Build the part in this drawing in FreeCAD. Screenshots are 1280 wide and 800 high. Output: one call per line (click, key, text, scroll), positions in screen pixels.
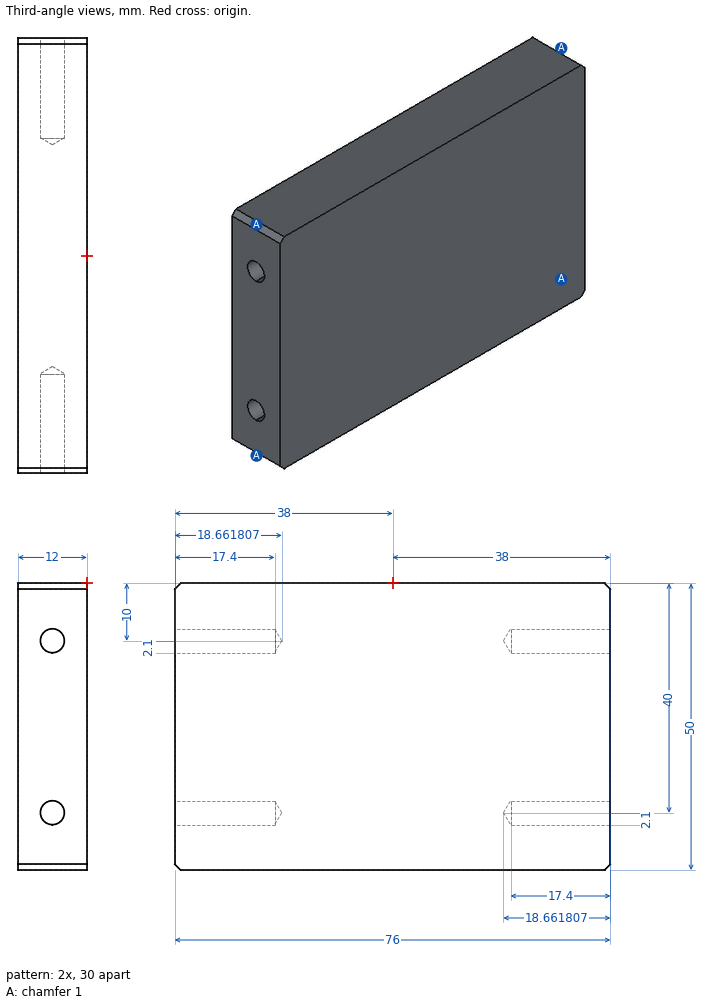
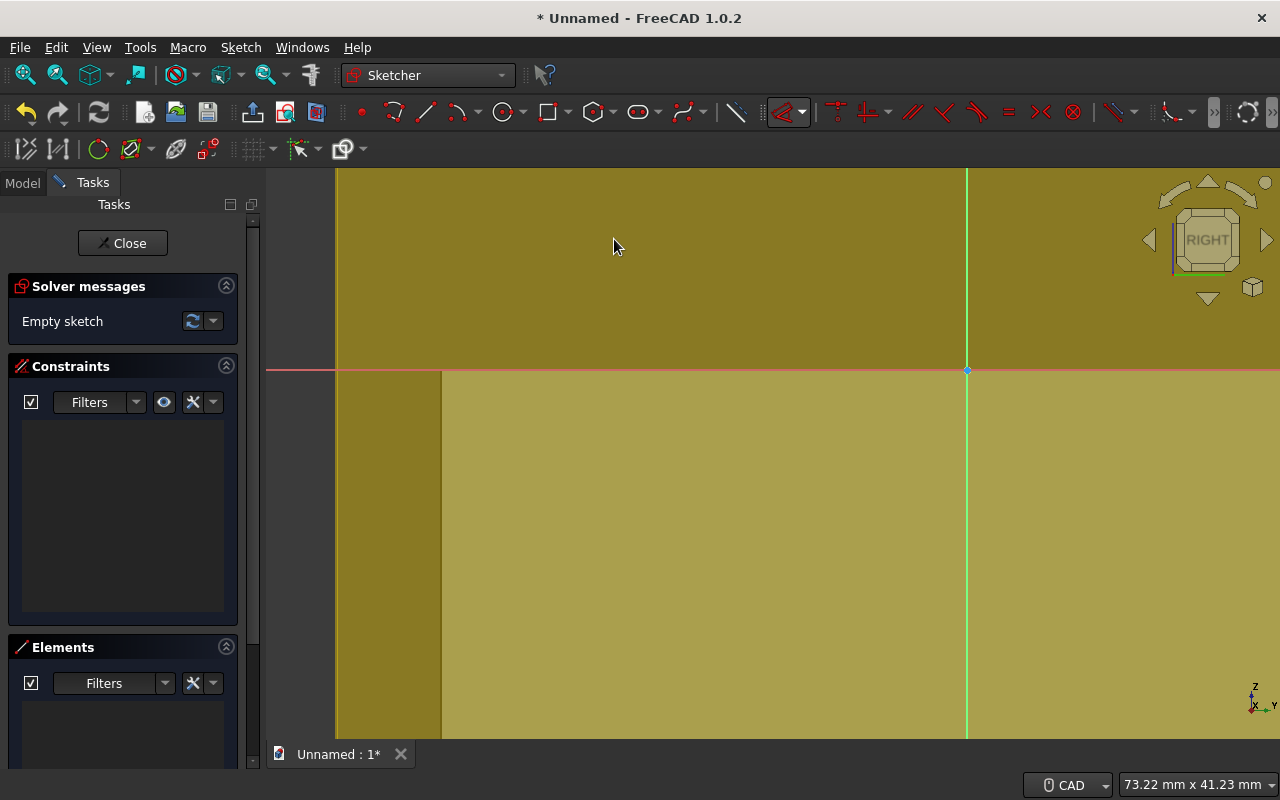
click(394, 112)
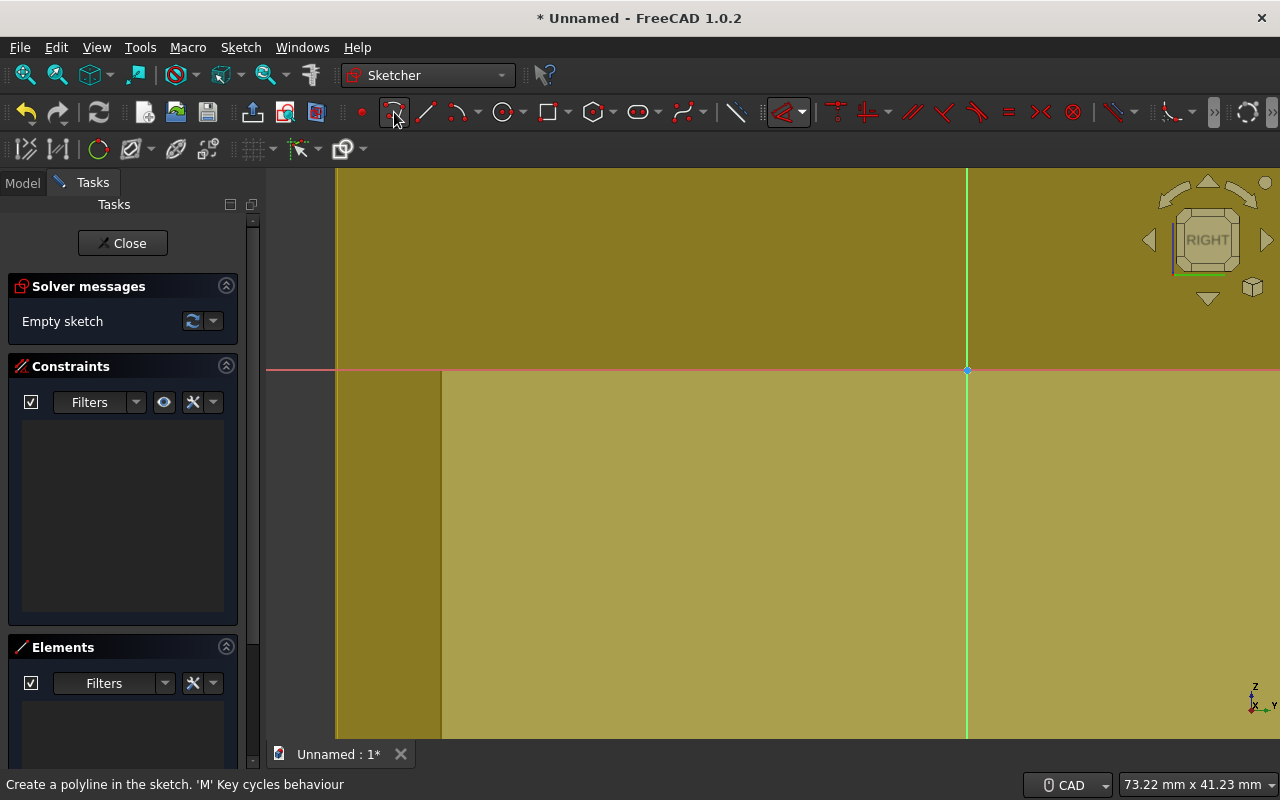
click(700, 508)
click(441, 508)
click(441, 538)
click(682, 538)
click(700, 509)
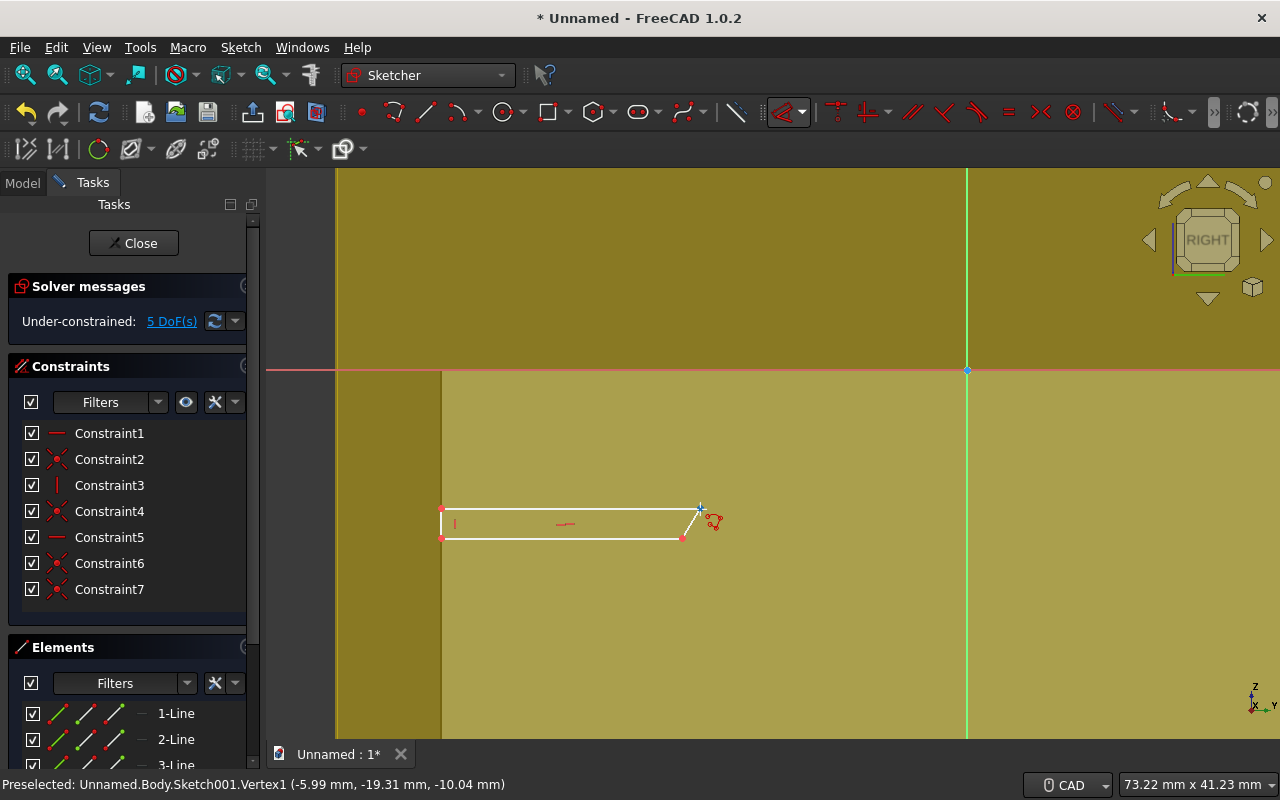
click(426, 112)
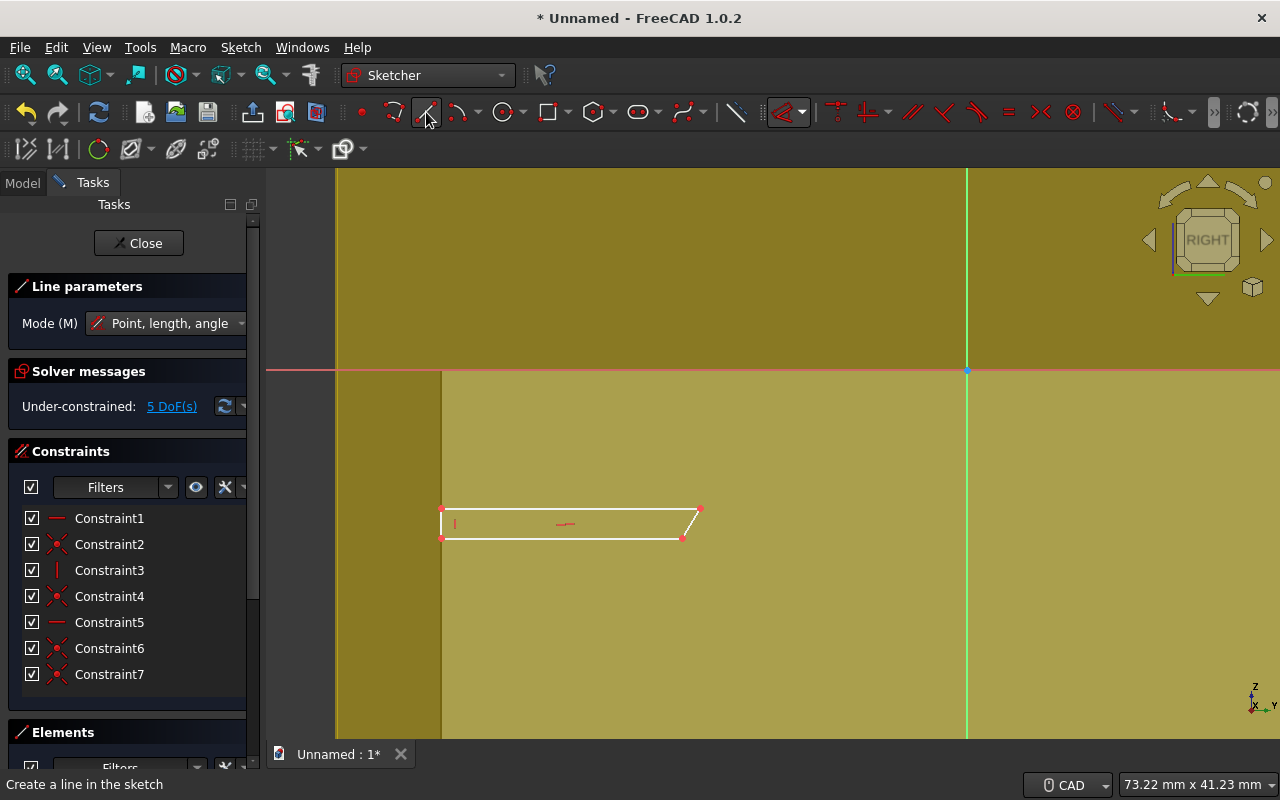
click(725, 508)
click(803, 508)
key(Escape)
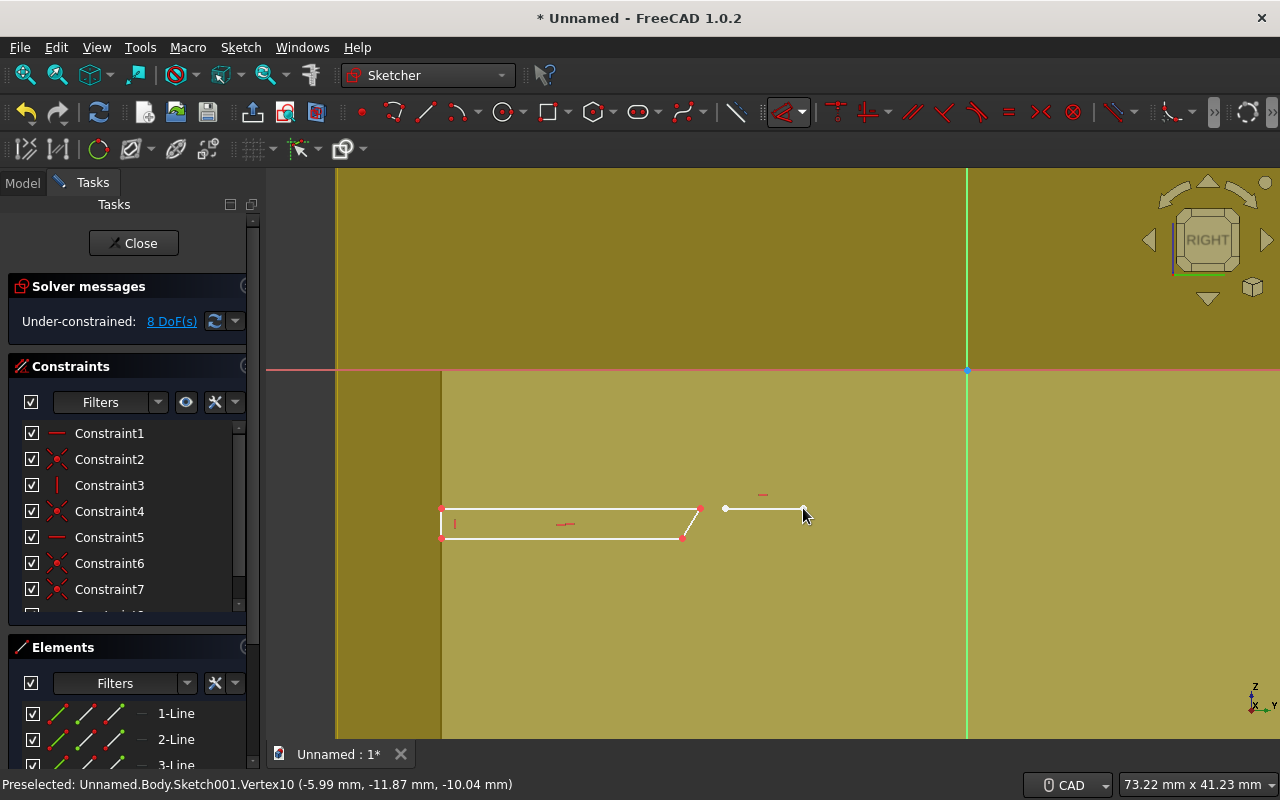
click(748, 509)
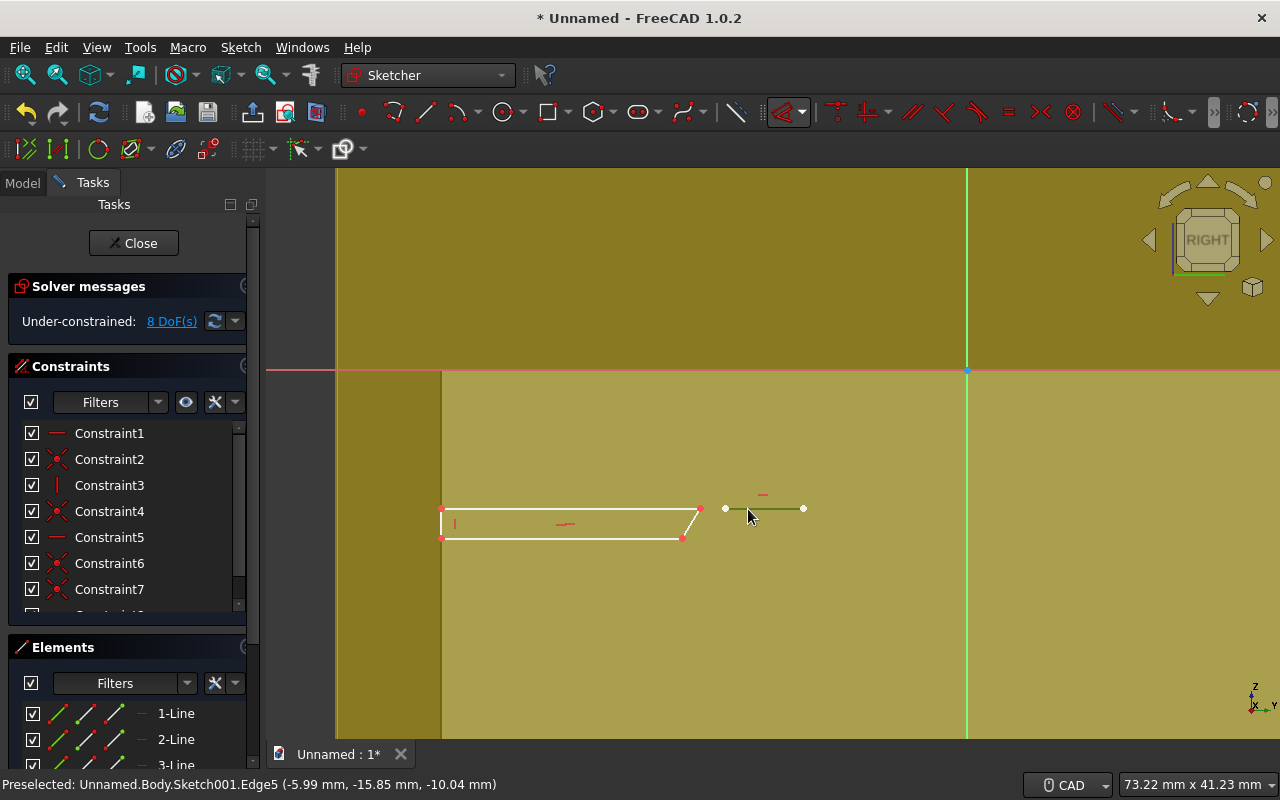
click(738, 112)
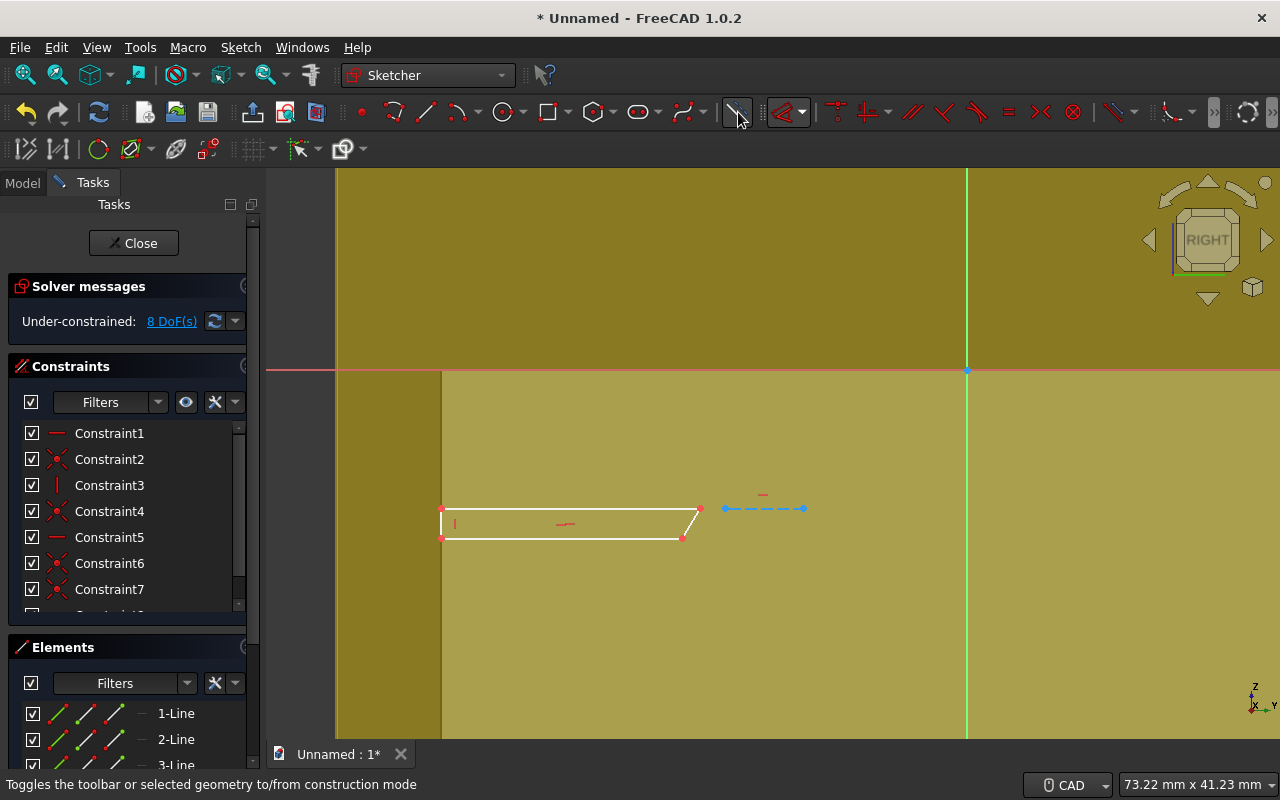
scroll(441, 521, up, 2)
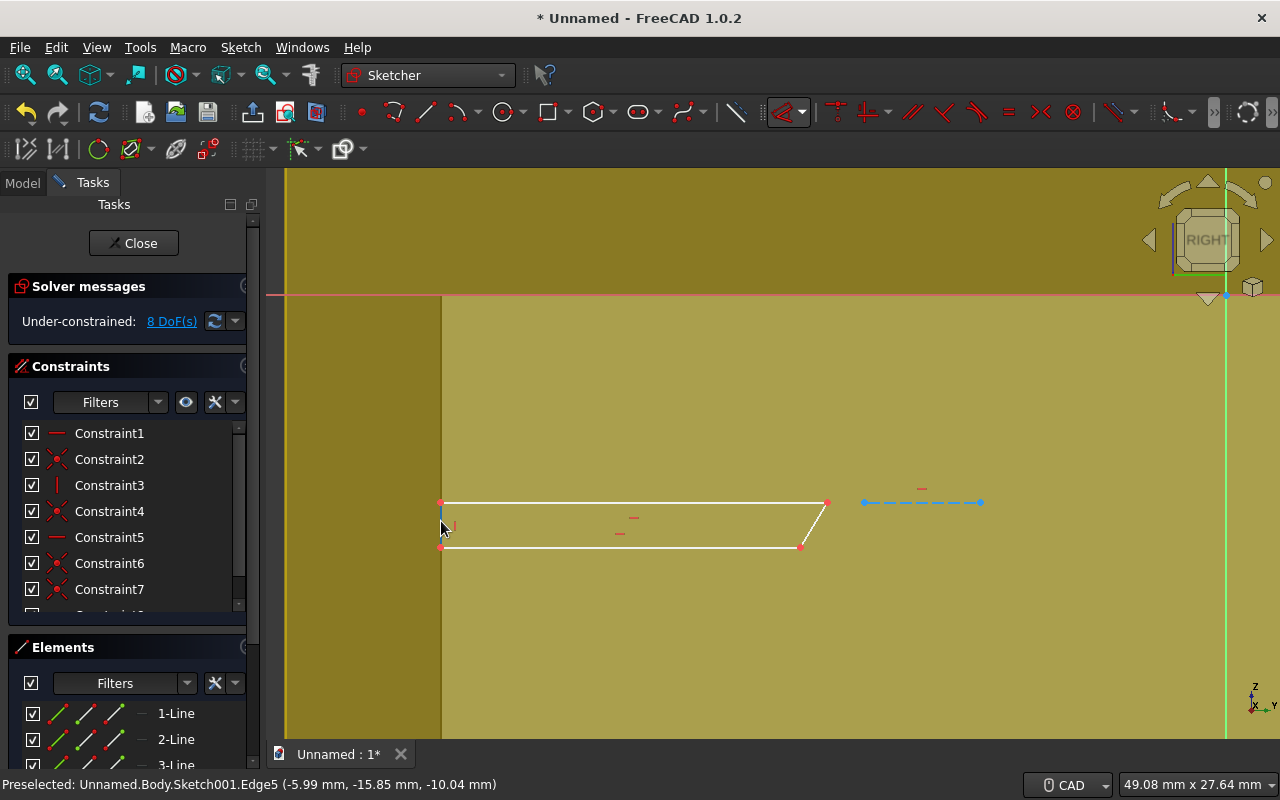
click(441, 521)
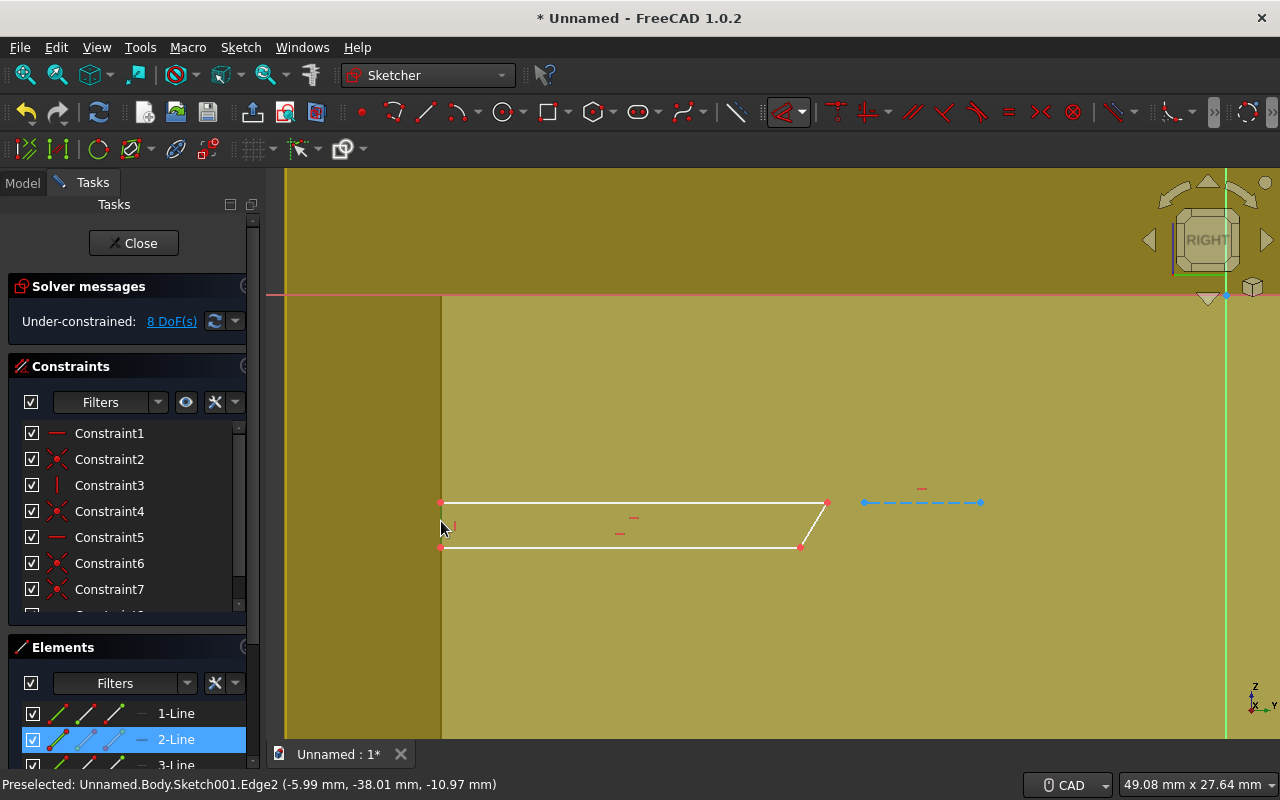
key(i)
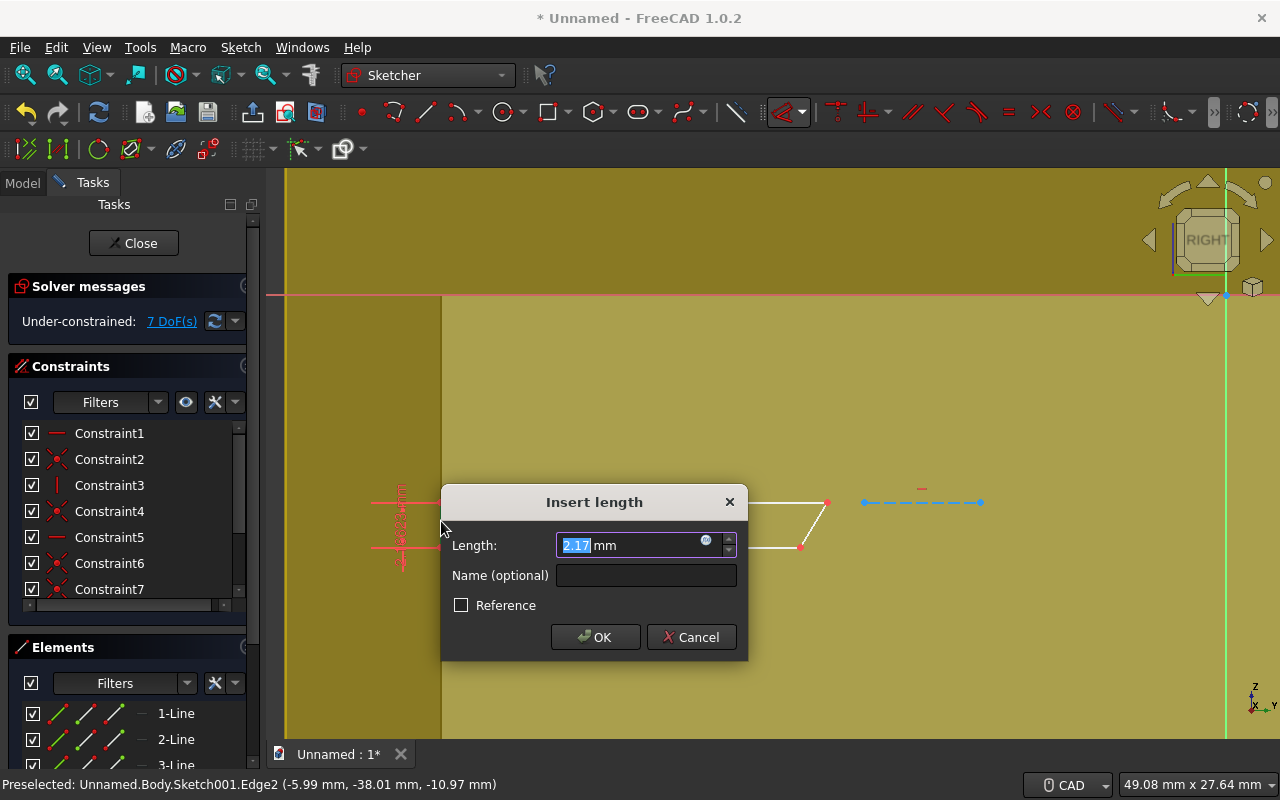
text(2.1)
key(Return)